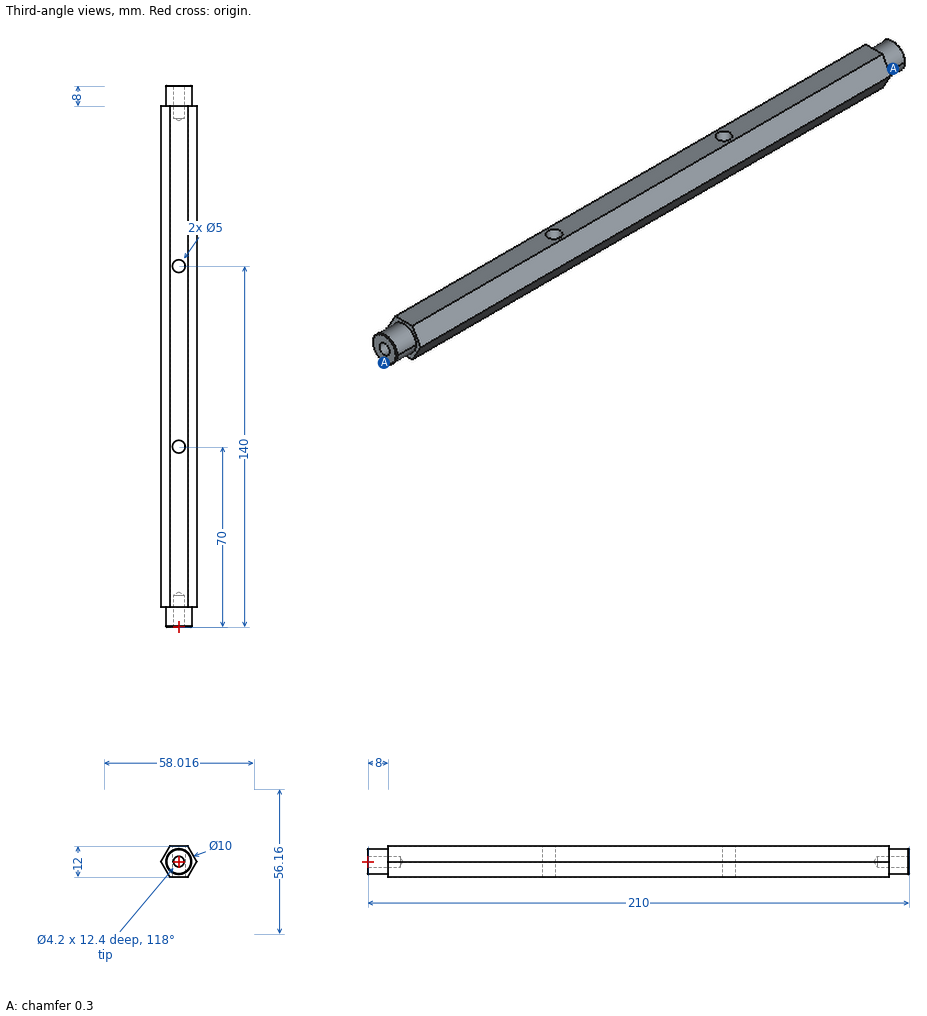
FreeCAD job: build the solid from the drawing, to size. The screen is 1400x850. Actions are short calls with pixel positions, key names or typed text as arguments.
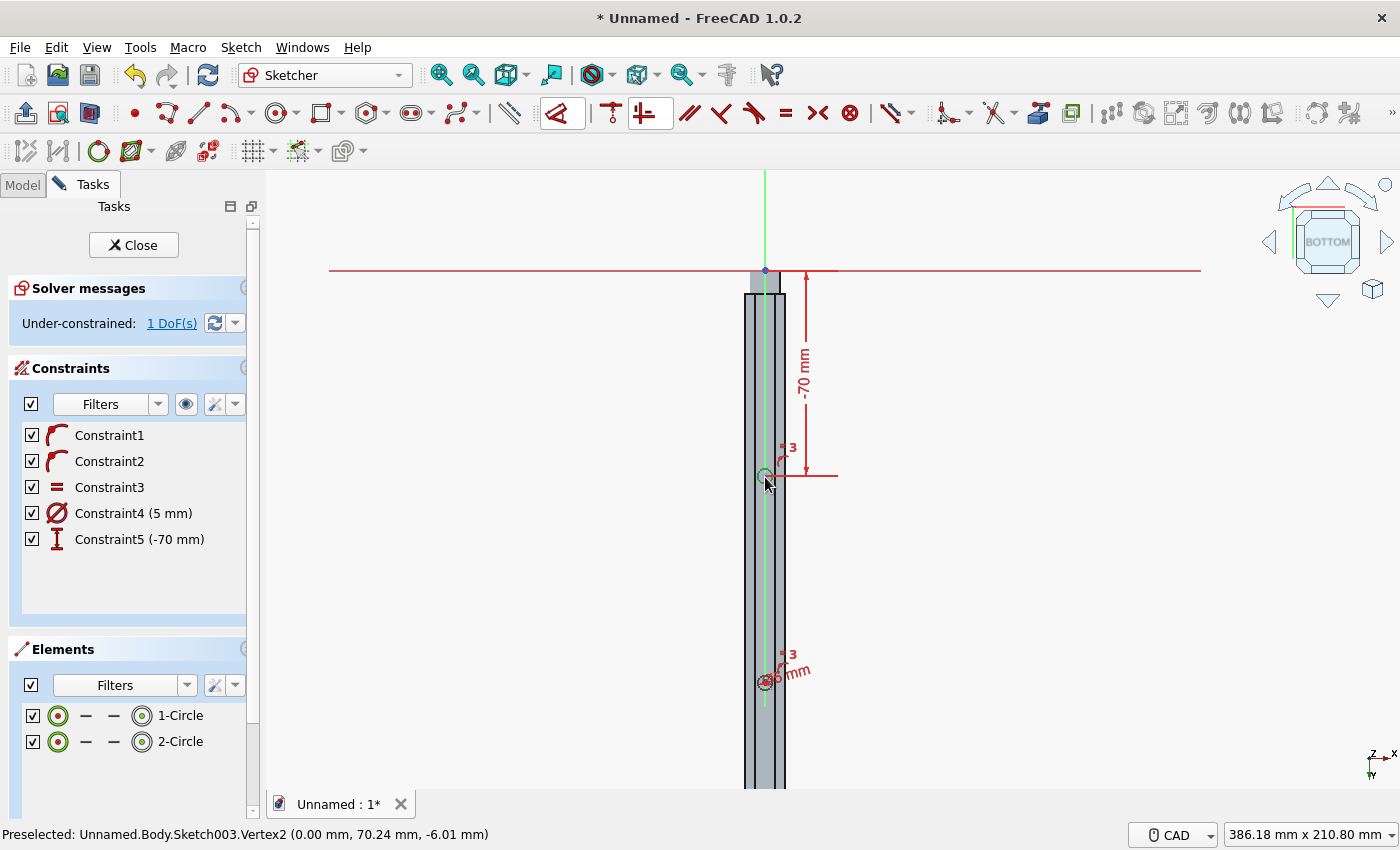
click(765, 683)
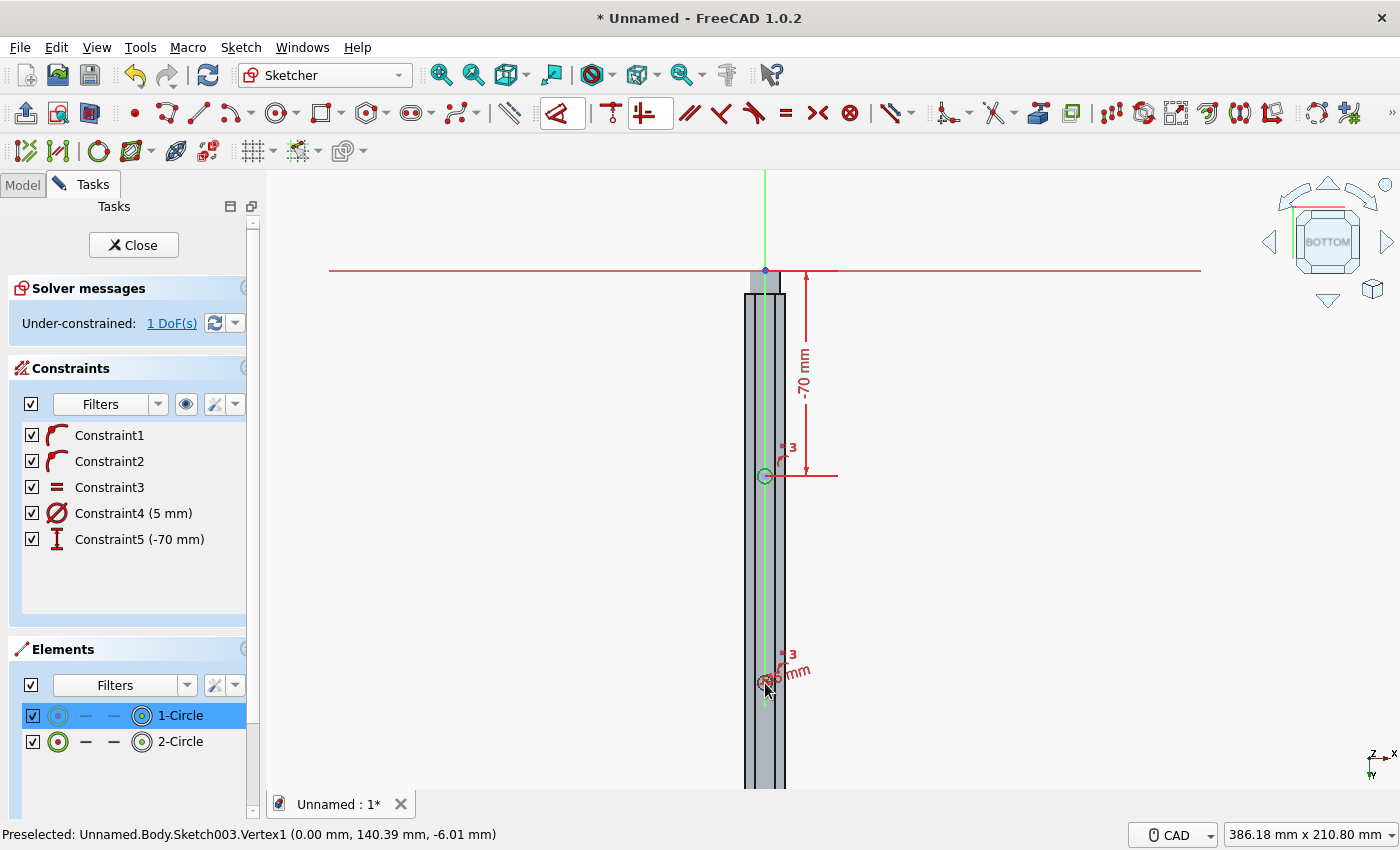
key(i)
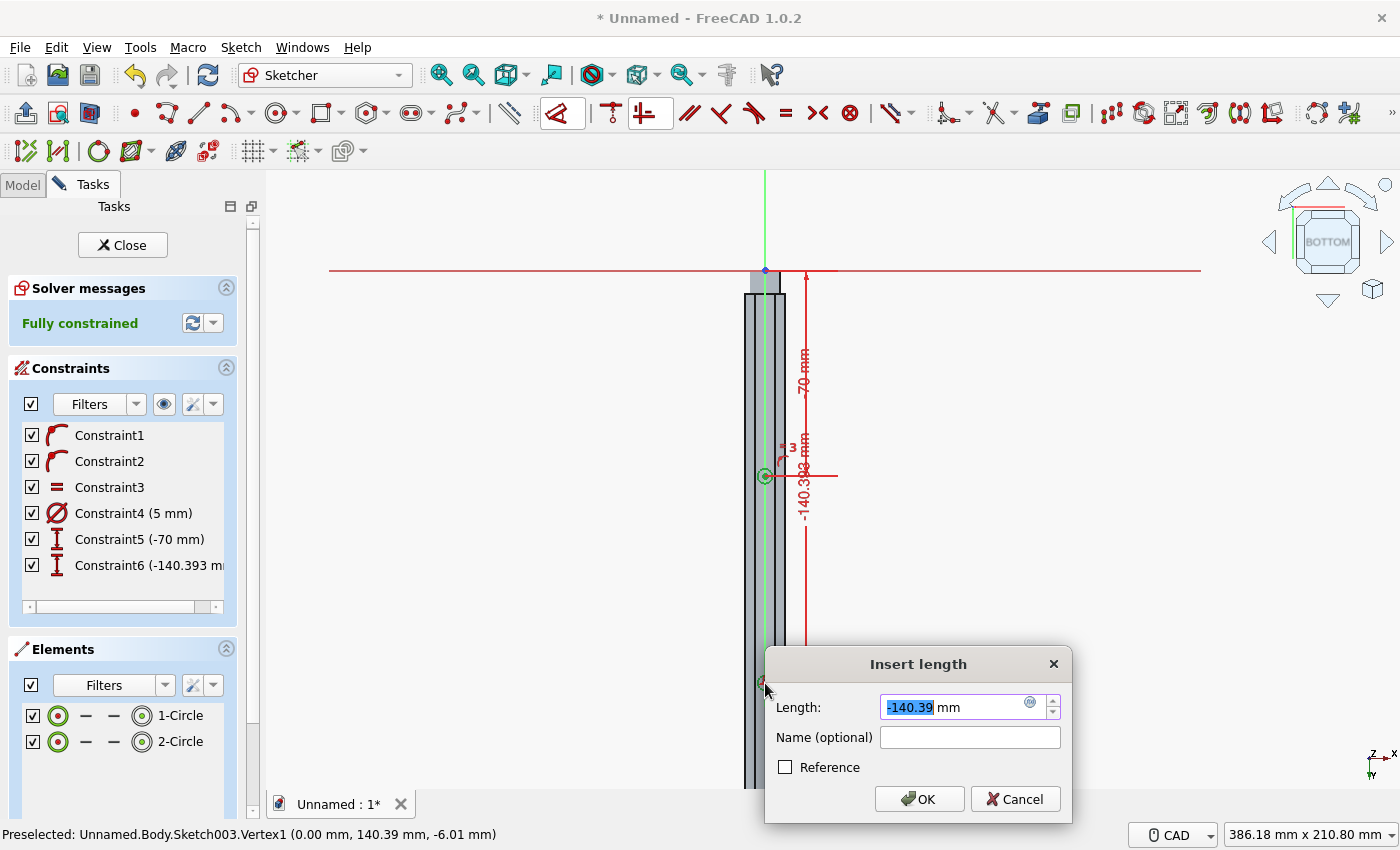
text(-140)
key(Return)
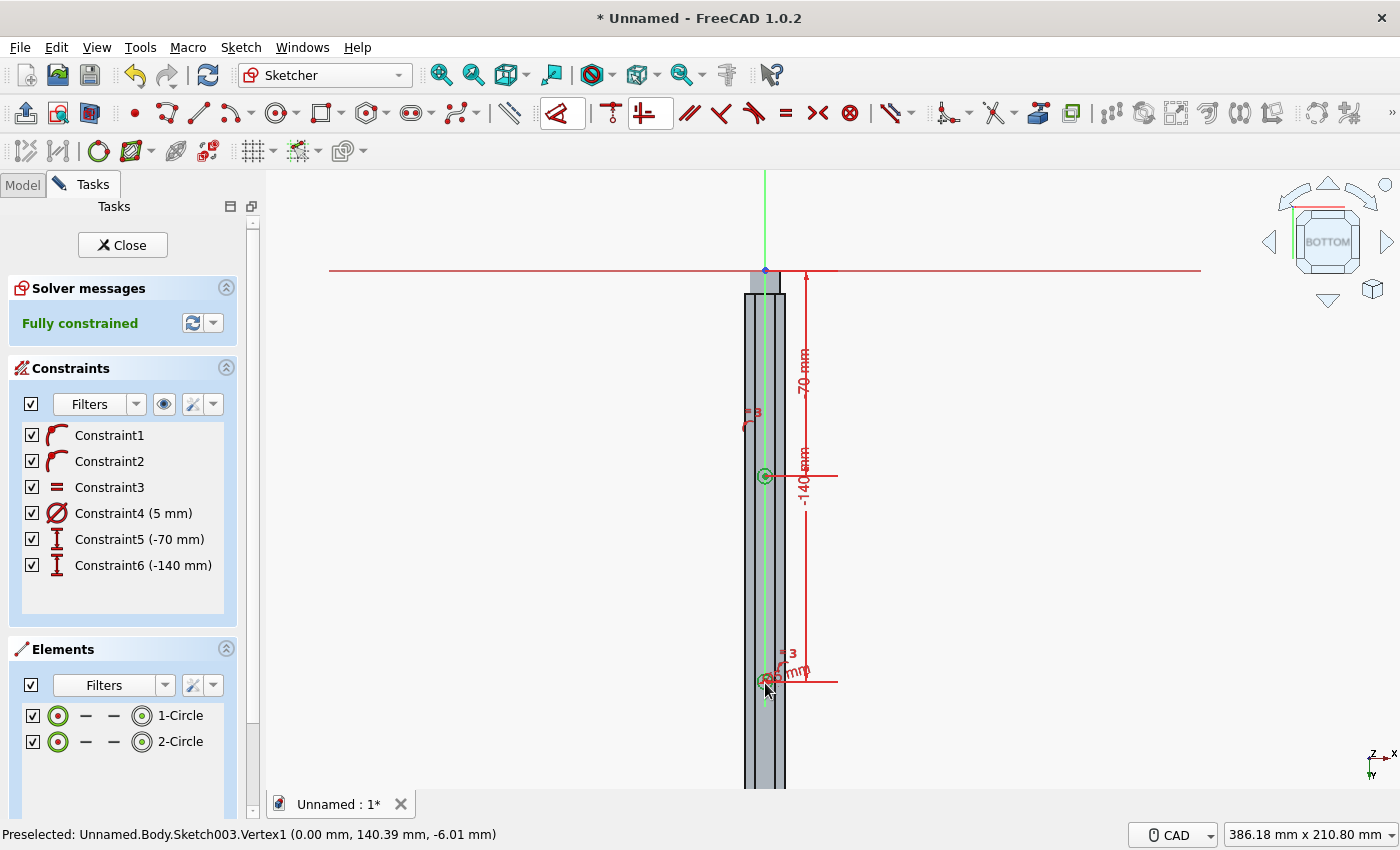
click(123, 245)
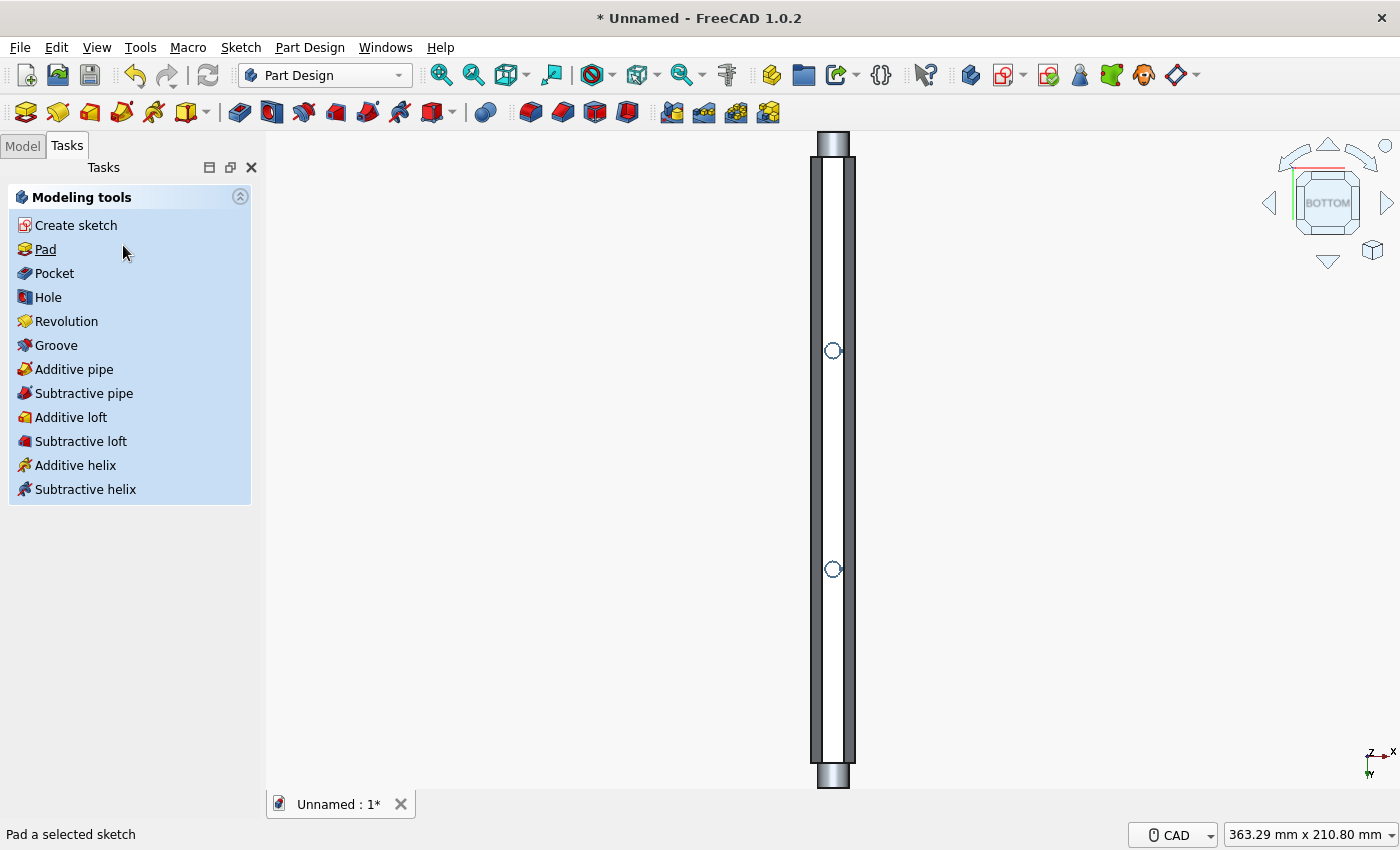
click(240, 112)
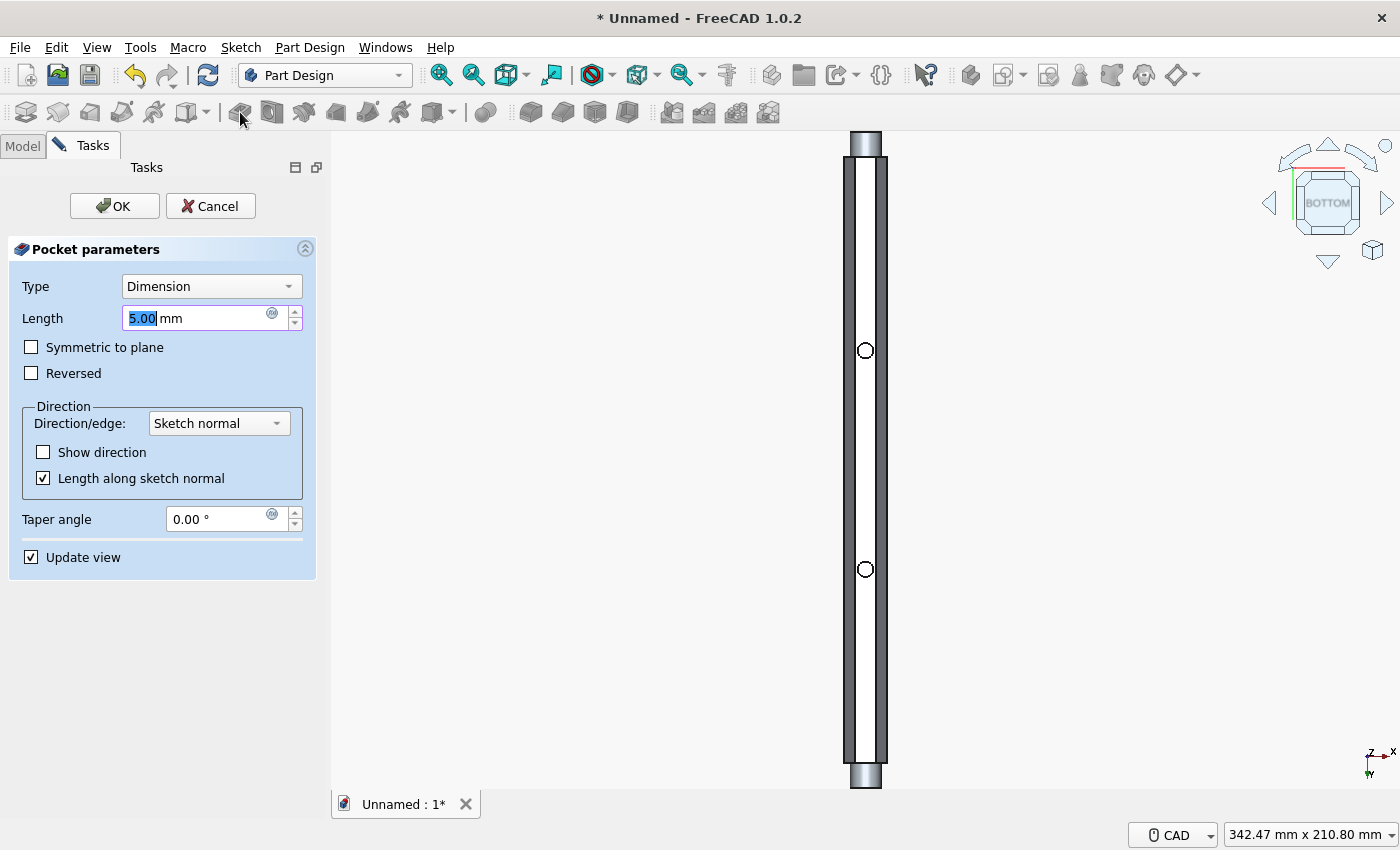
click(212, 286)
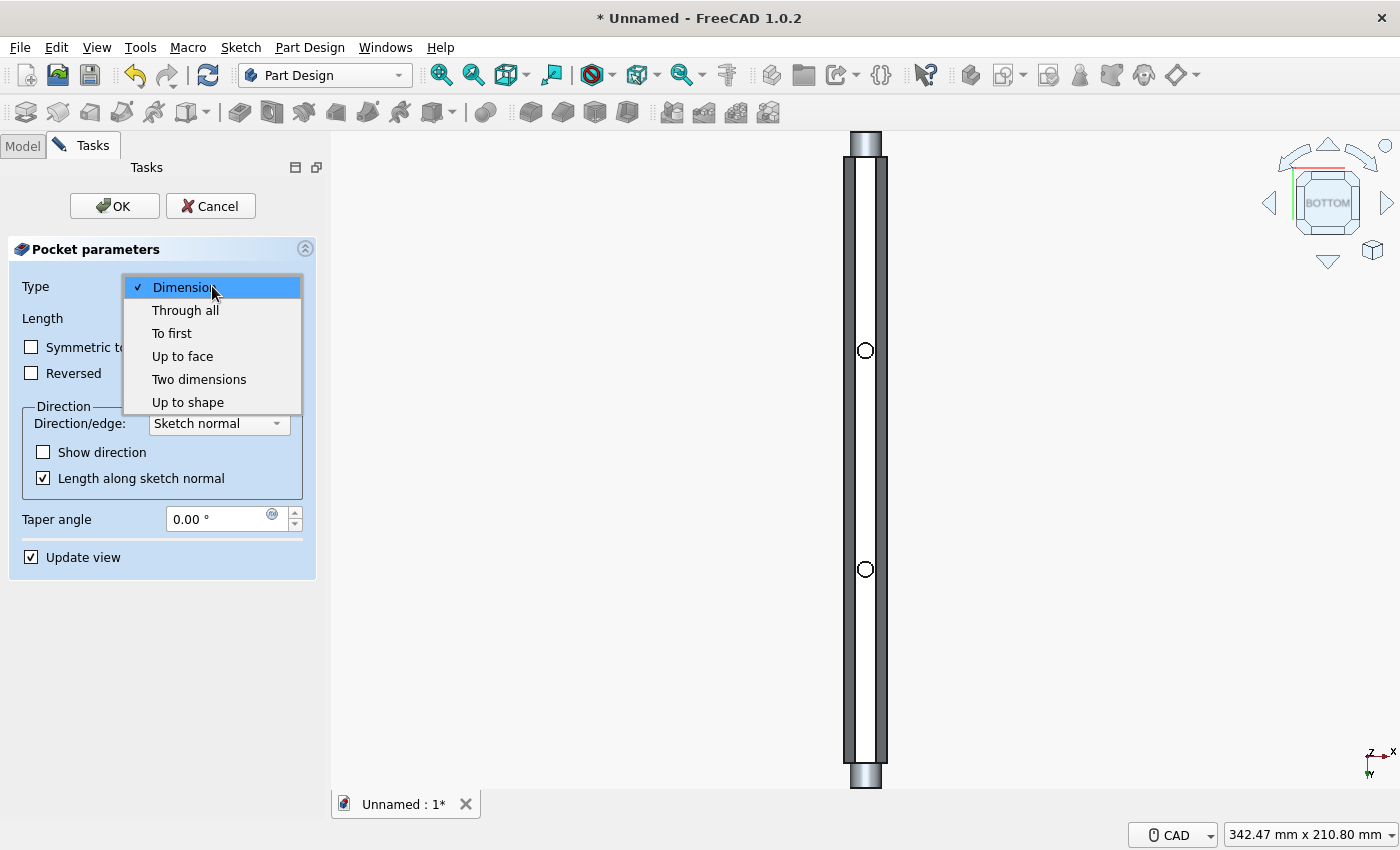
click(212, 310)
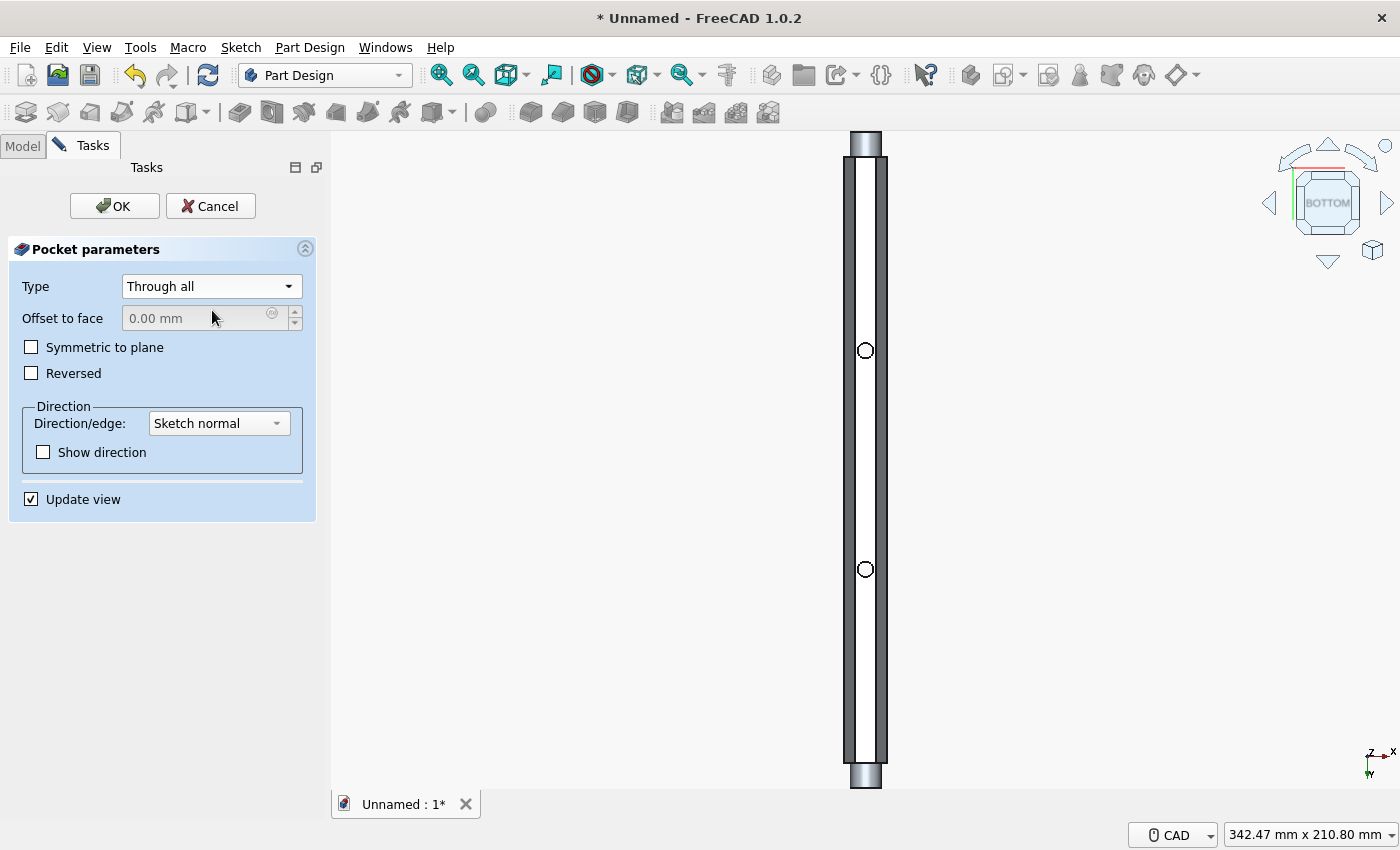
click(115, 206)